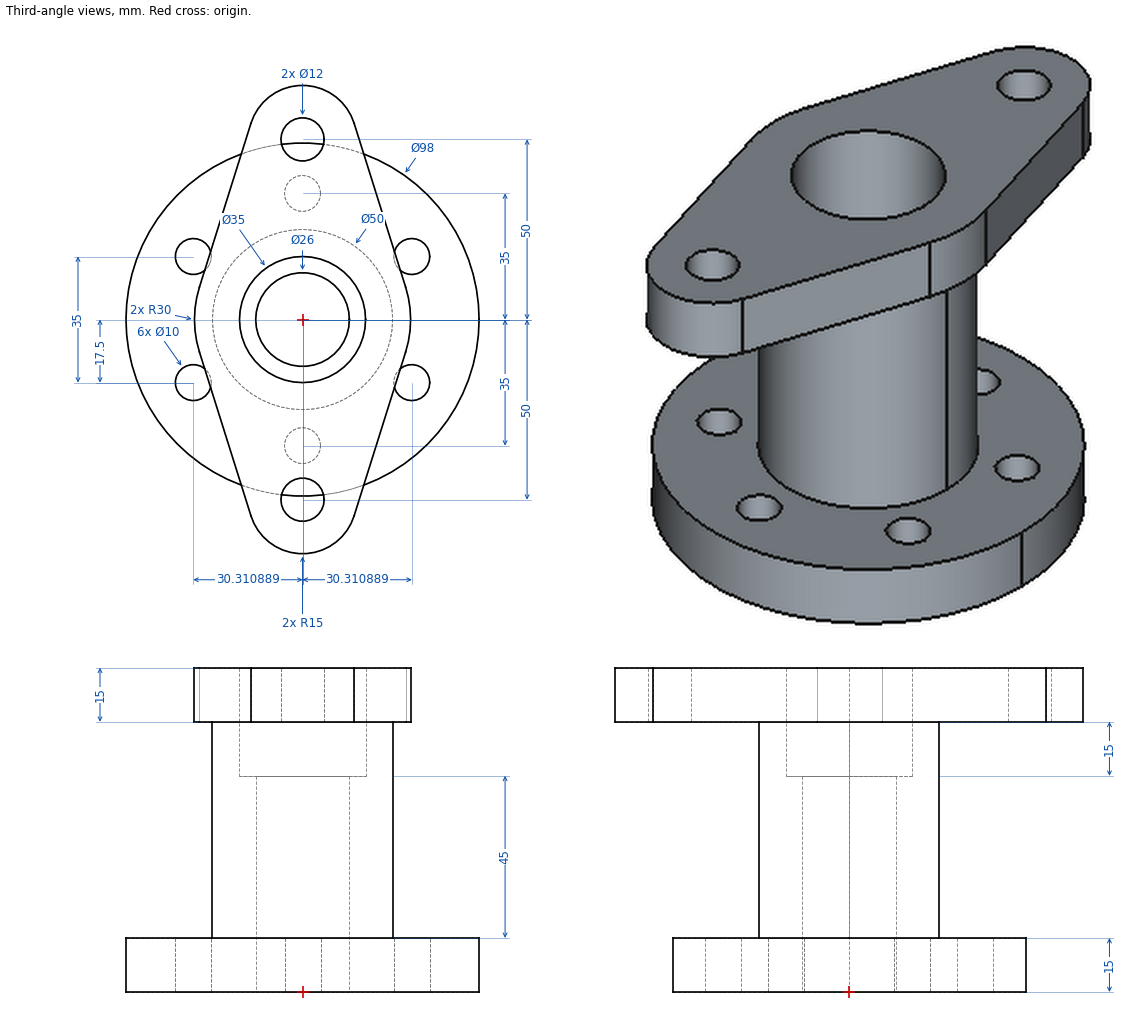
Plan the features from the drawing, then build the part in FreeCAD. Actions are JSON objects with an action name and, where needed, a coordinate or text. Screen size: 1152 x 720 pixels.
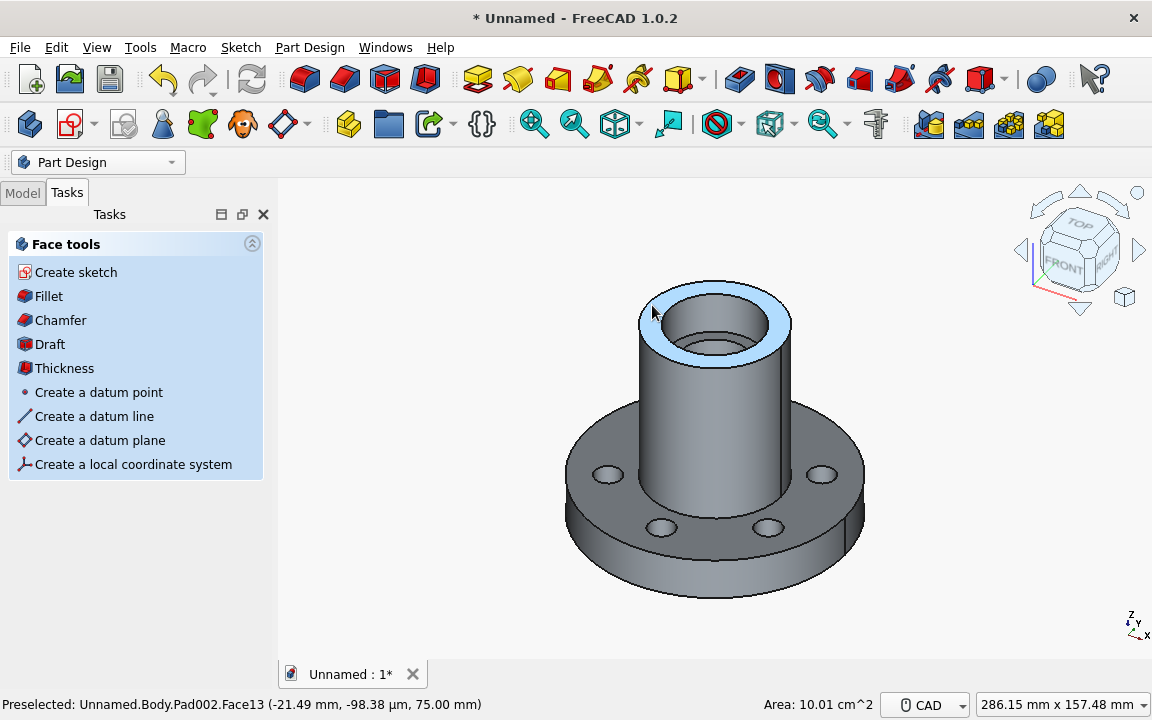
{"action": "left_click", "coordinate": [70, 124]}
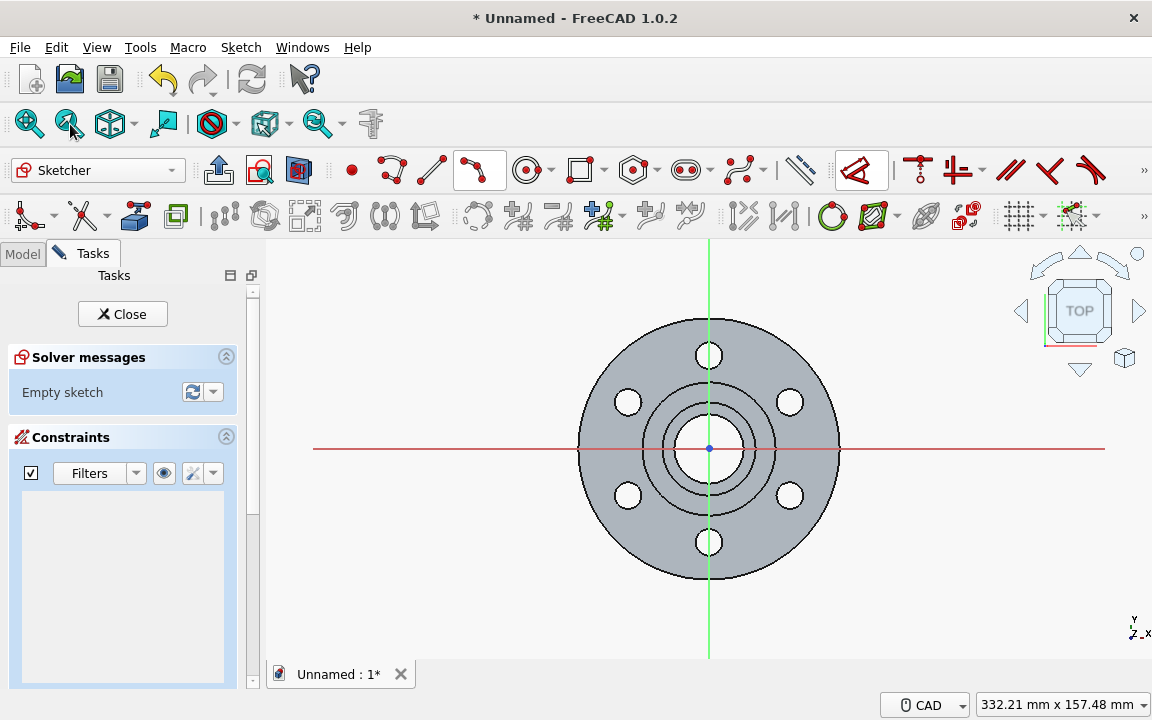
{"action": "scroll", "coordinate": [331, 449], "scroll_direction": "down", "scroll_amount": 1}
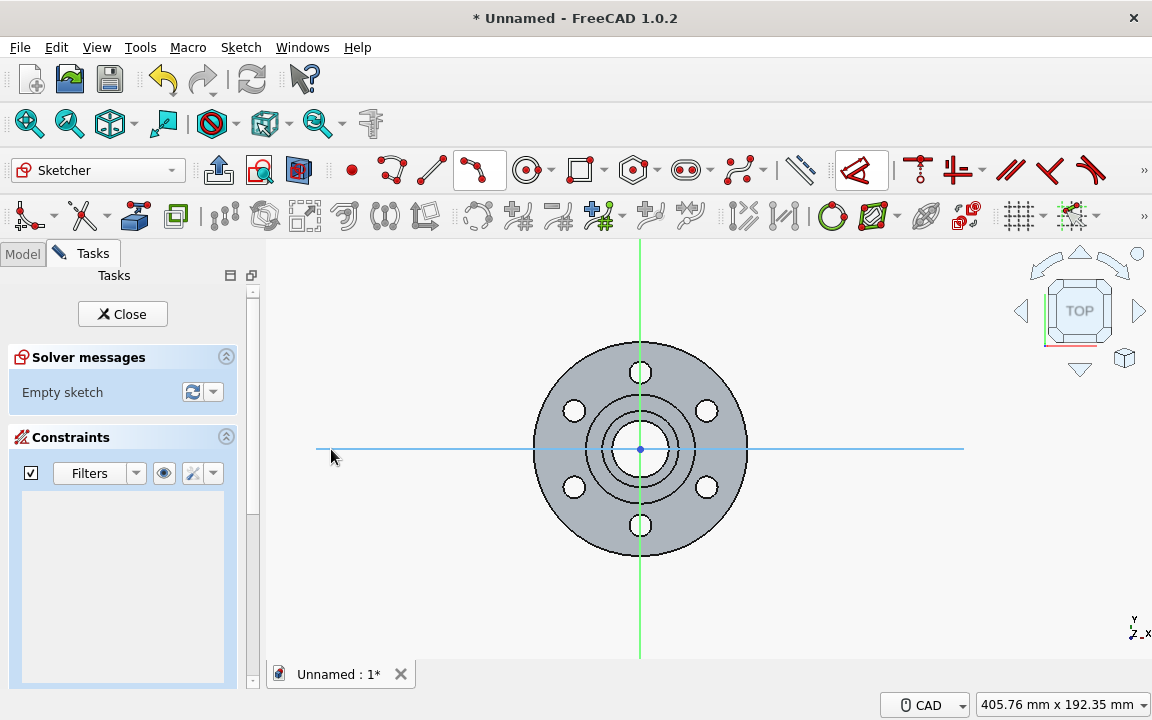
{"action": "key", "text": "g l"}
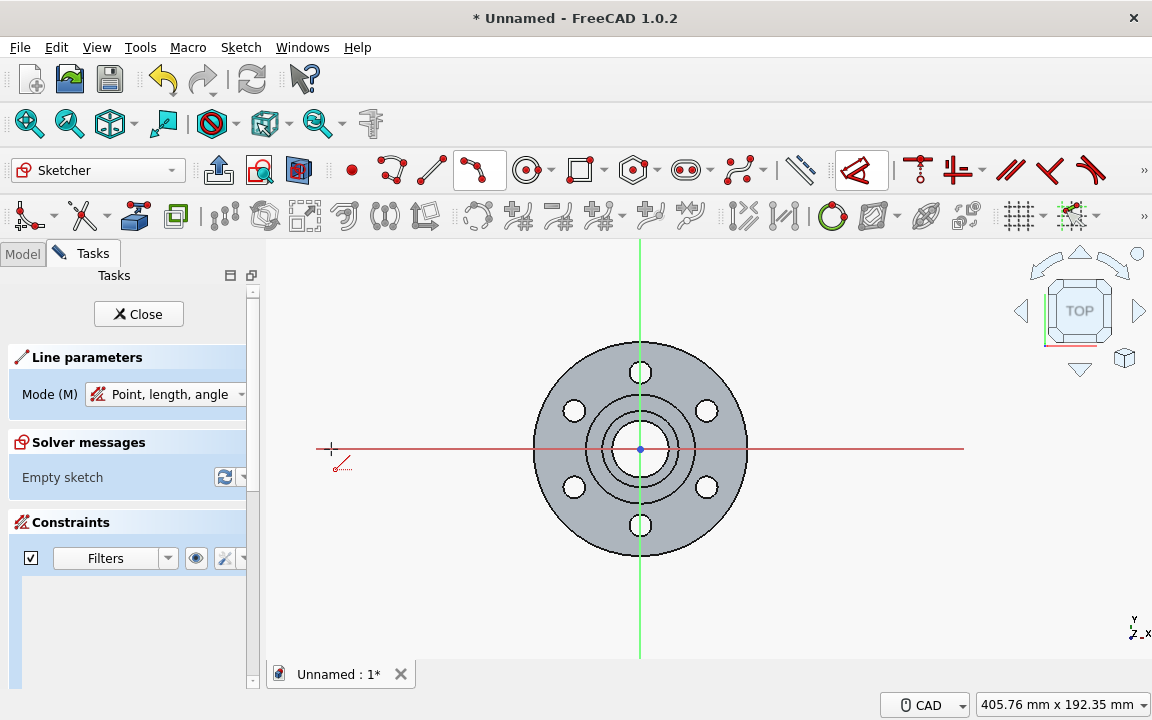
{"action": "left_click", "coordinate": [609, 330]}
{"action": "left_click", "coordinate": [578, 429]}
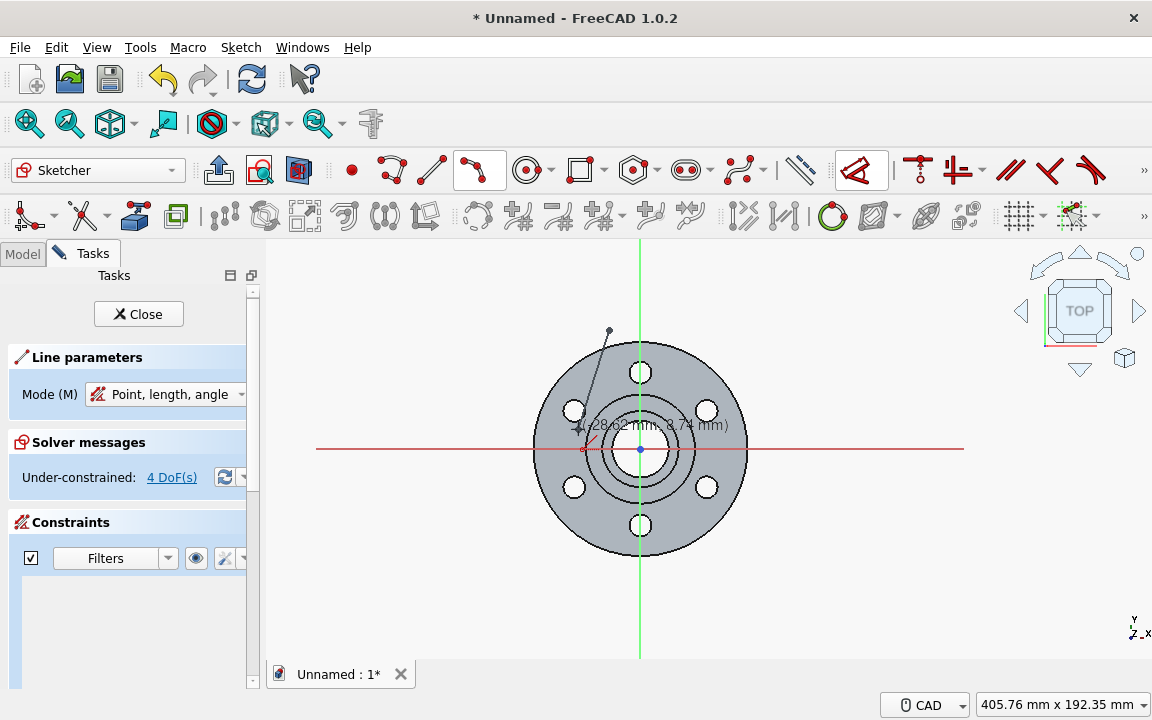
{"action": "left_click", "coordinate": [578, 469]}
{"action": "left_click", "coordinate": [609, 568]}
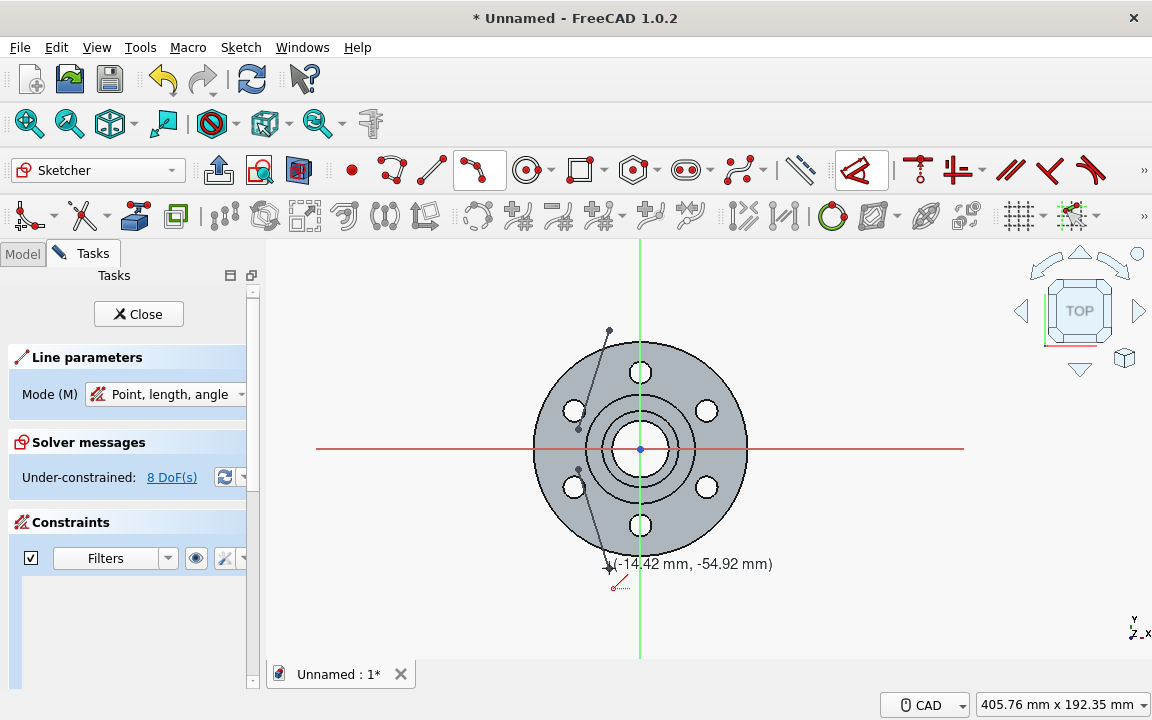
{"action": "left_click", "coordinate": [672, 568]}
{"action": "left_click", "coordinate": [703, 469]}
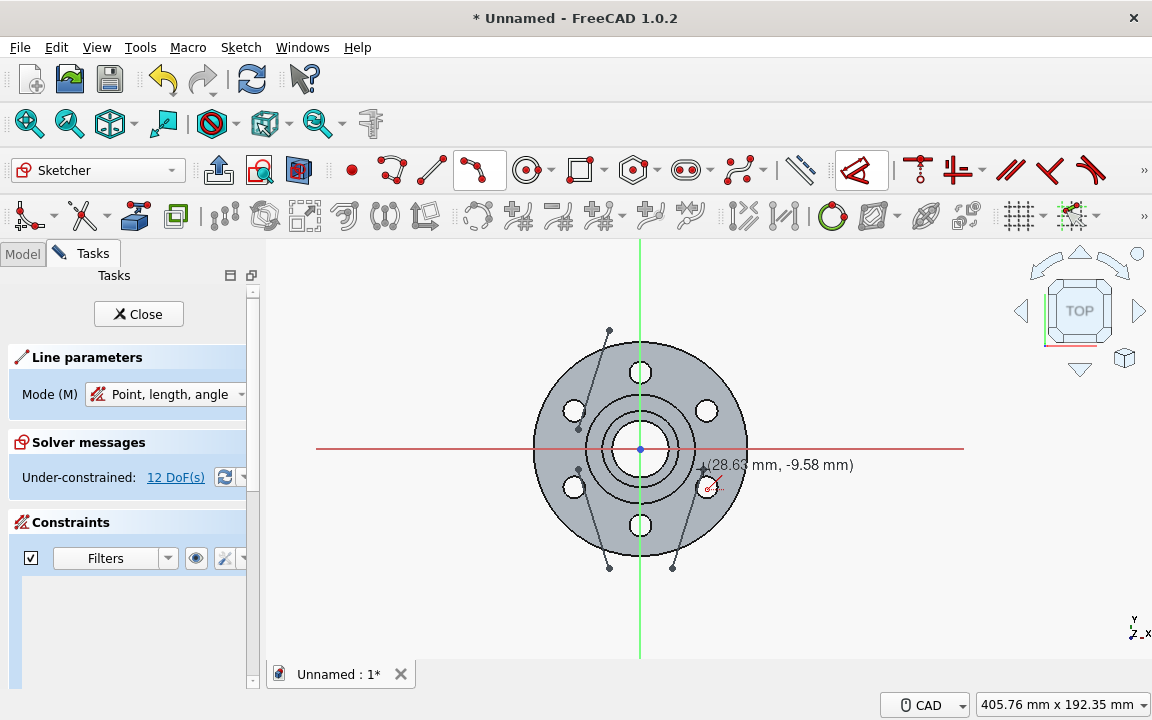
{"action": "left_click", "coordinate": [703, 429]}
{"action": "left_click", "coordinate": [672, 330]}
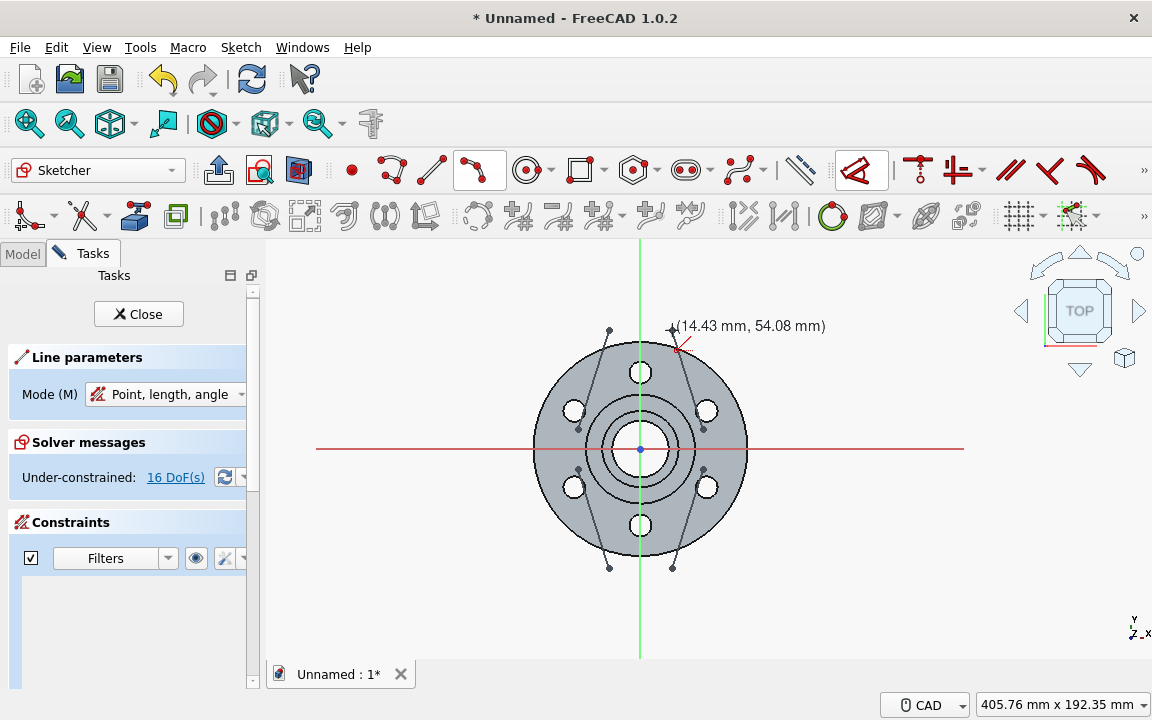
{"action": "left_click", "coordinate": [474, 170]}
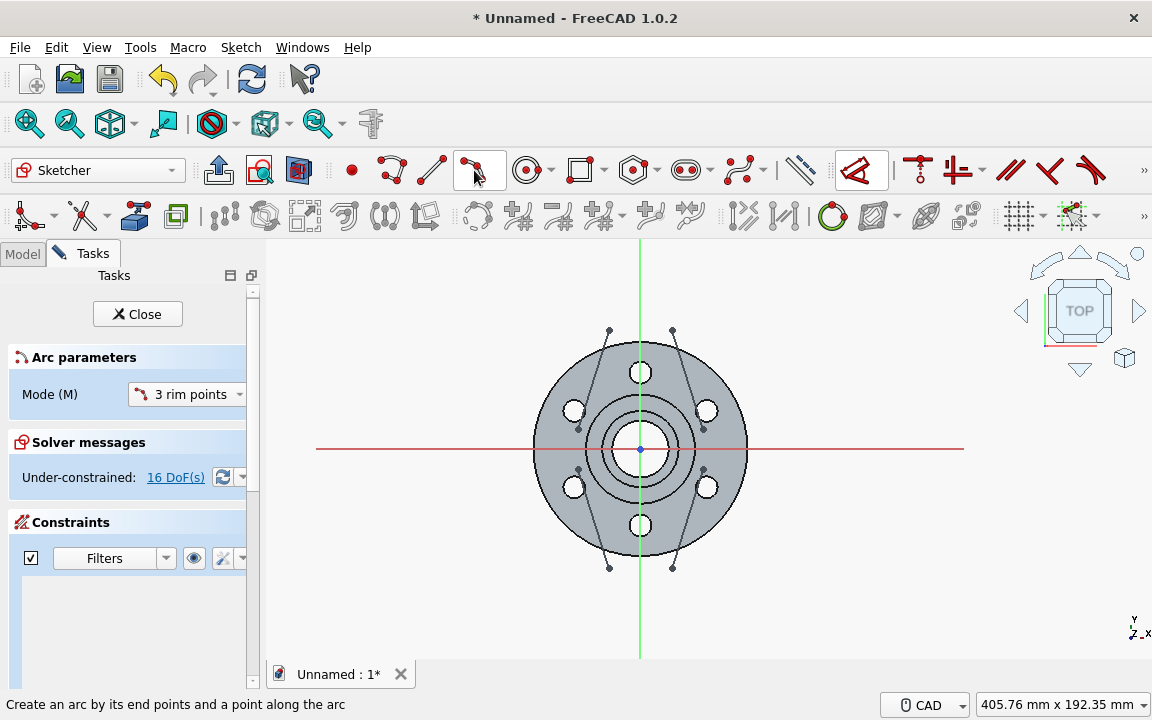
{"action": "left_click", "coordinate": [578, 430]}
{"action": "left_click", "coordinate": [578, 470]}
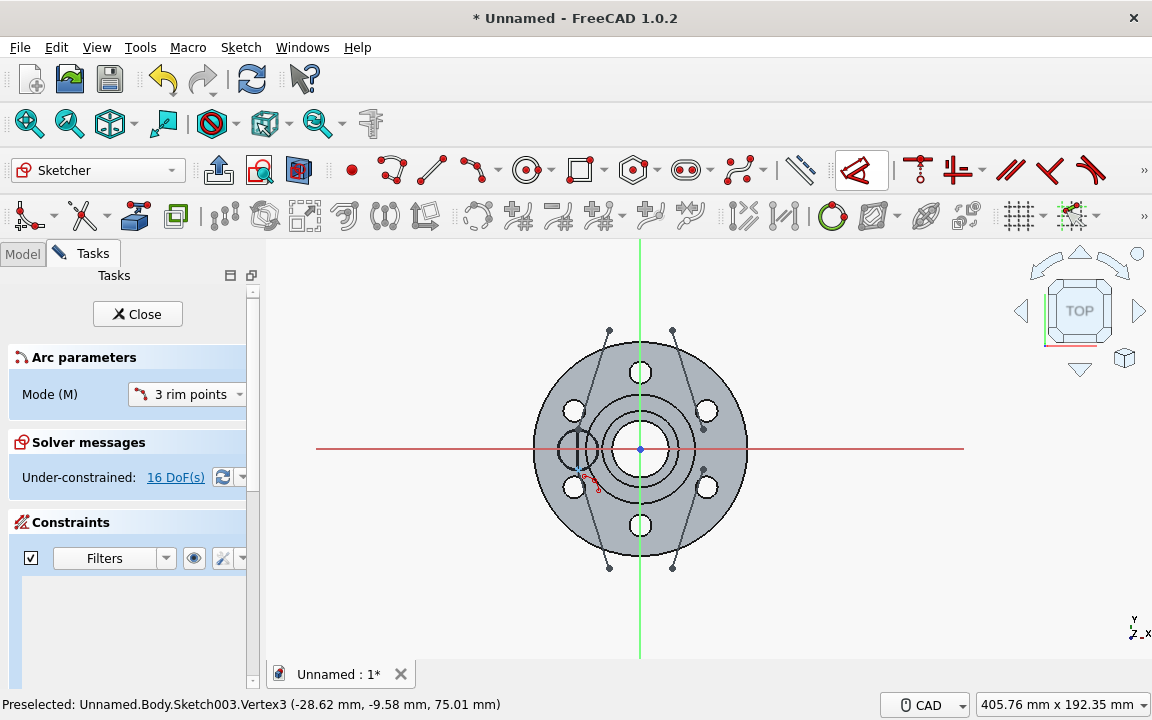
{"action": "scroll", "coordinate": [575, 445], "scroll_direction": "up", "scroll_amount": 9}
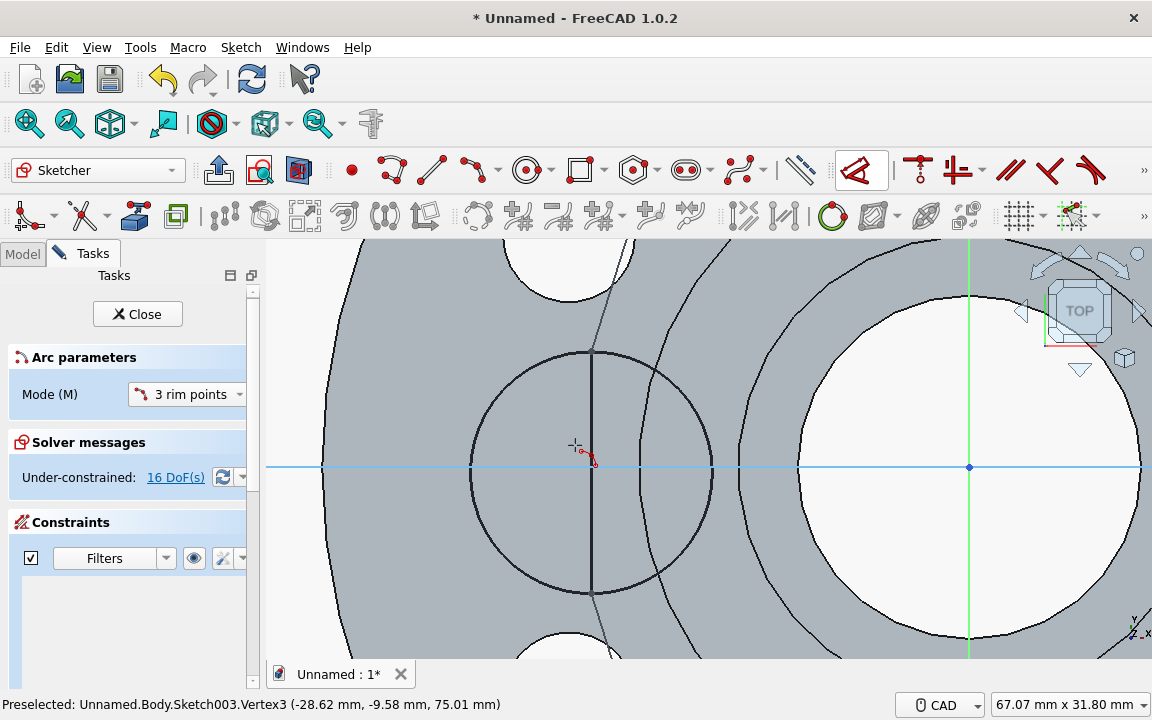
{"action": "left_click", "coordinate": [574, 443]}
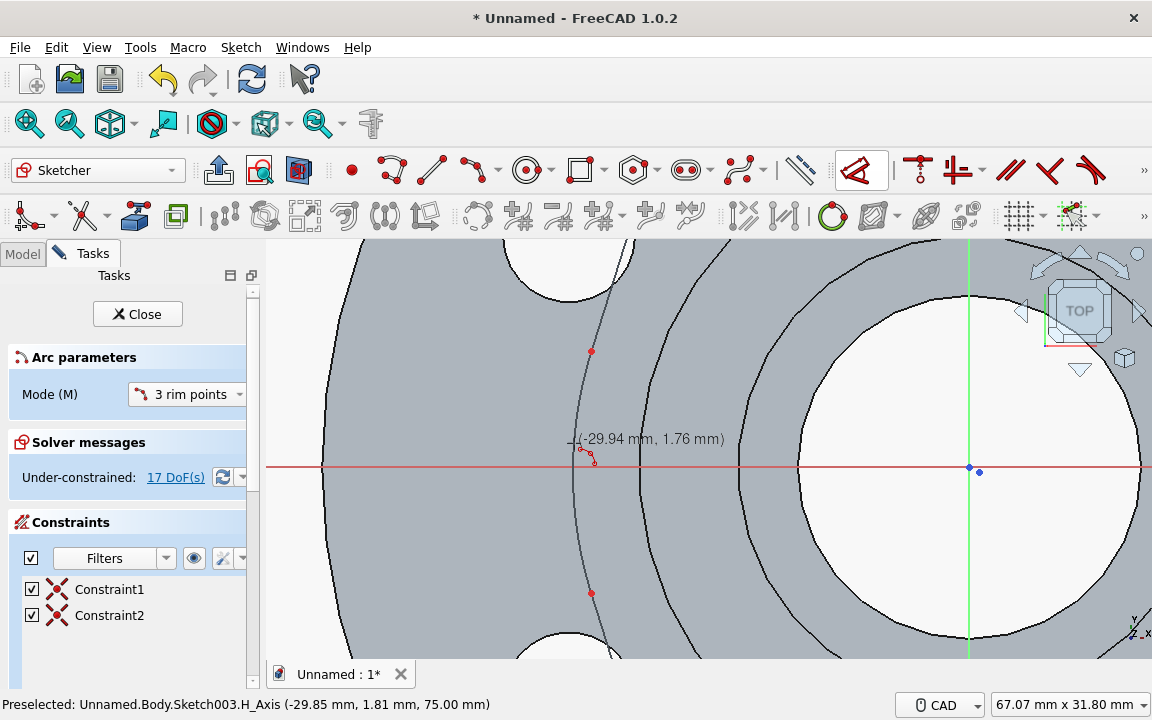
{"action": "scroll", "coordinate": [575, 445], "scroll_direction": "down", "scroll_amount": 9}